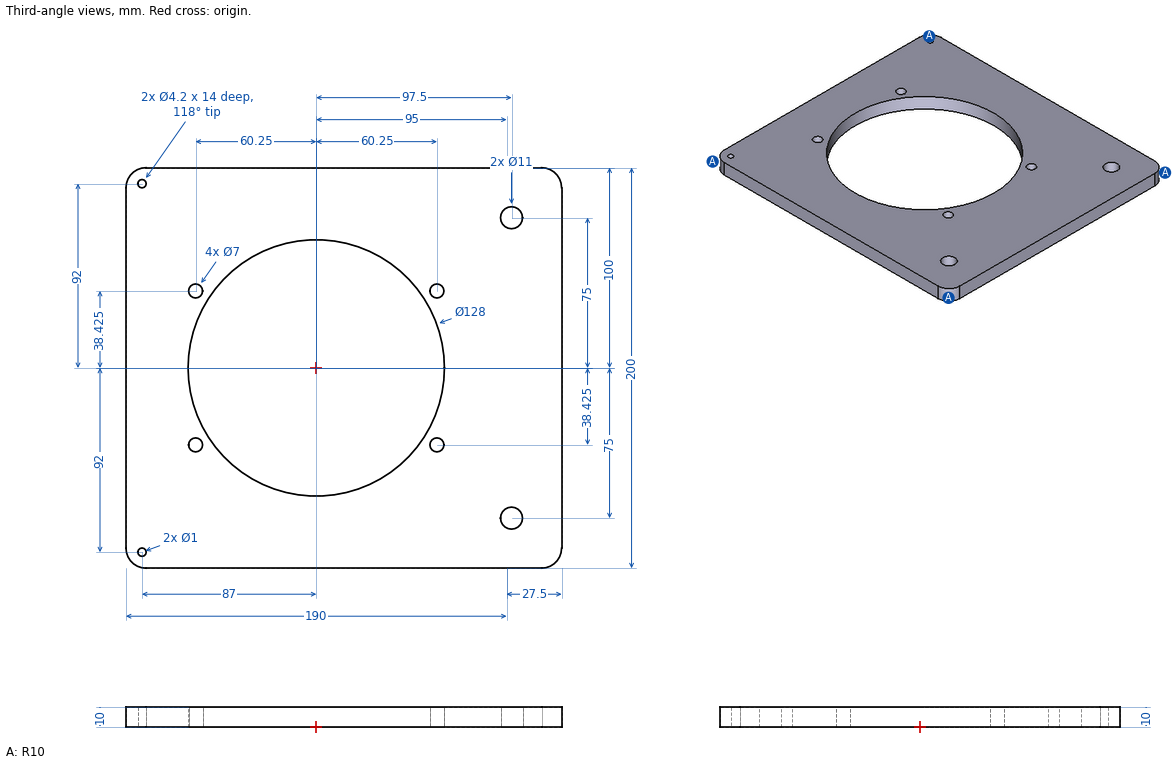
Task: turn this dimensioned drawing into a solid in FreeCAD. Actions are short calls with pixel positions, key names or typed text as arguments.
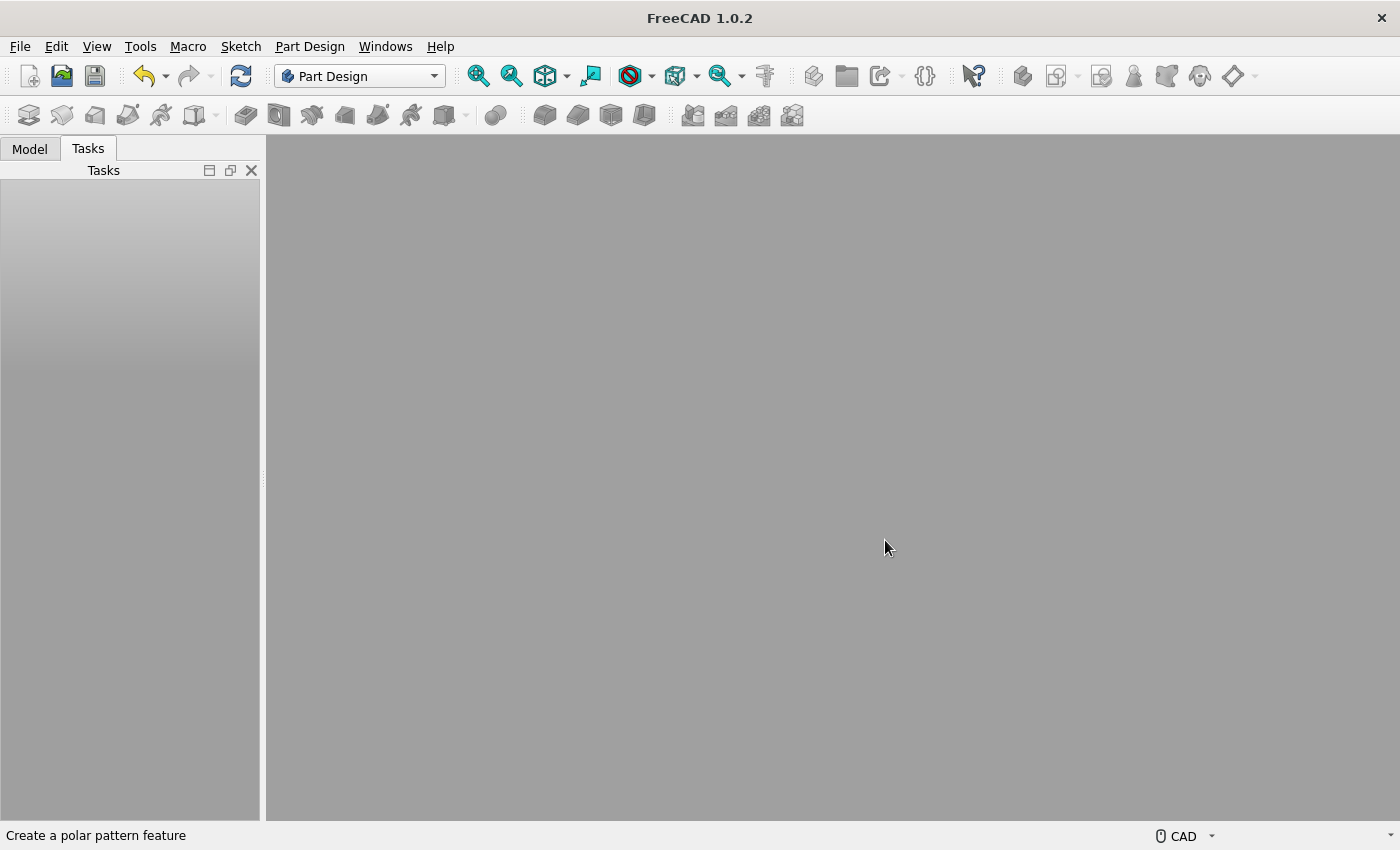
click(29, 76)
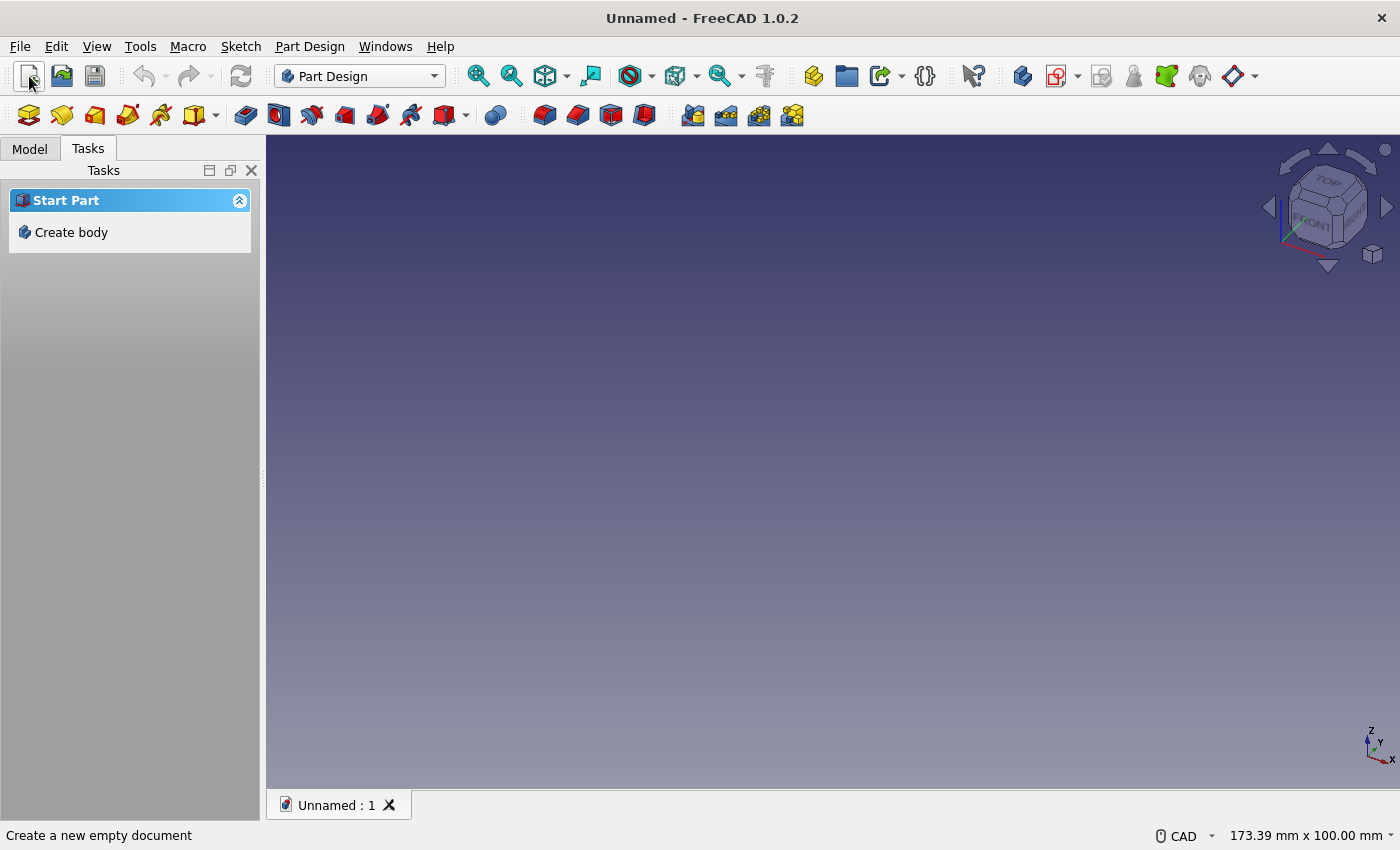
click(1056, 76)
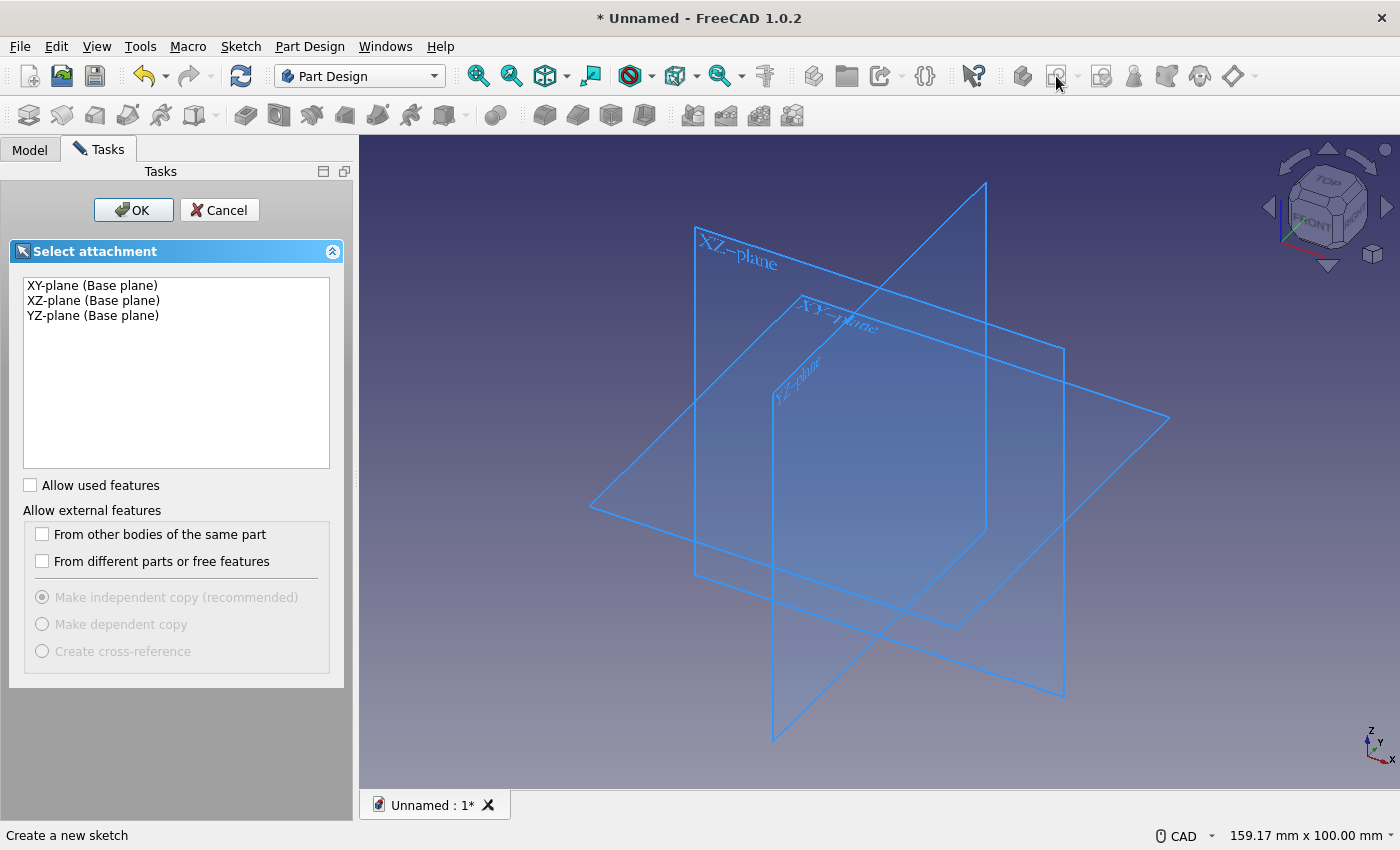
click(84, 286)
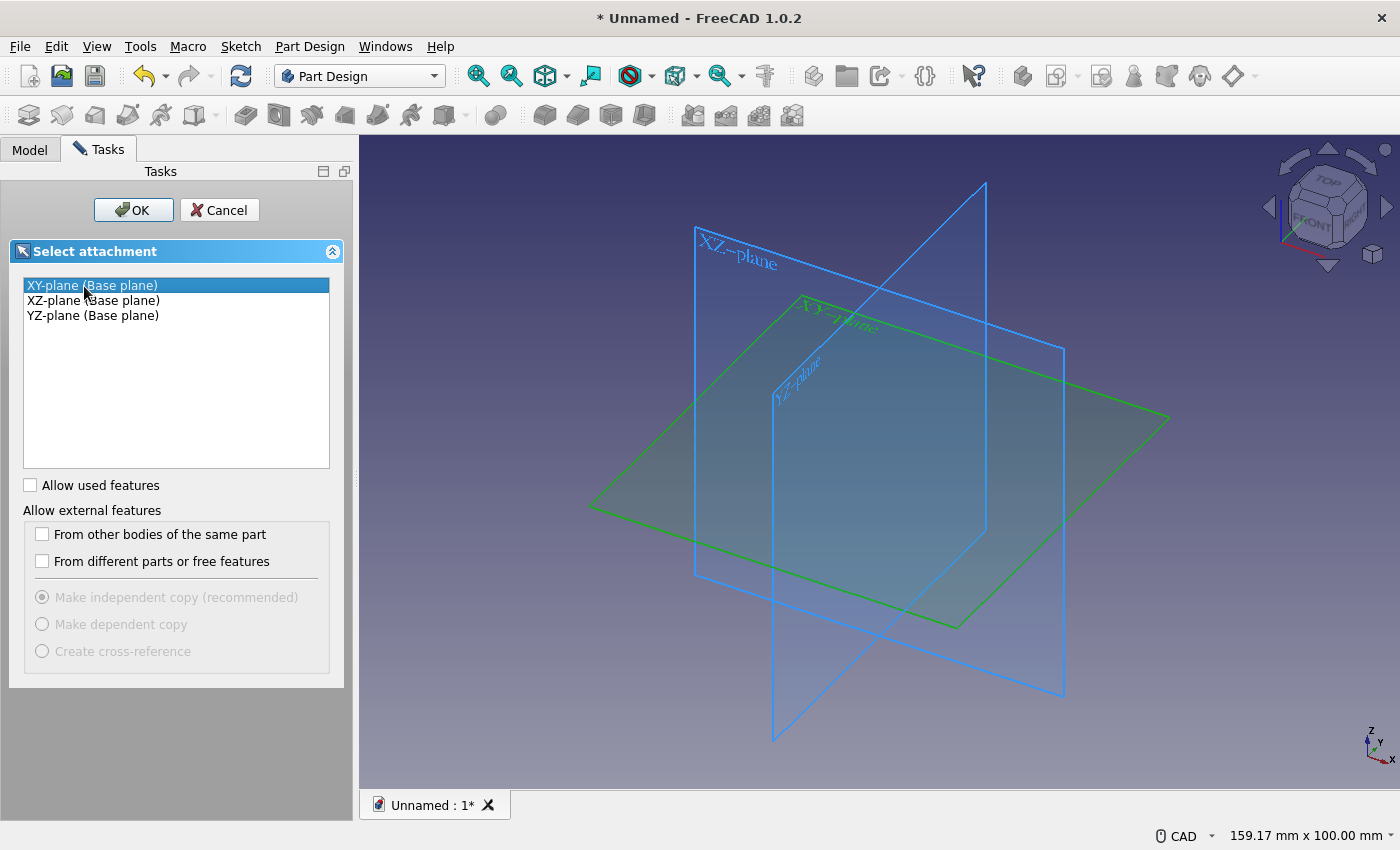
click(134, 210)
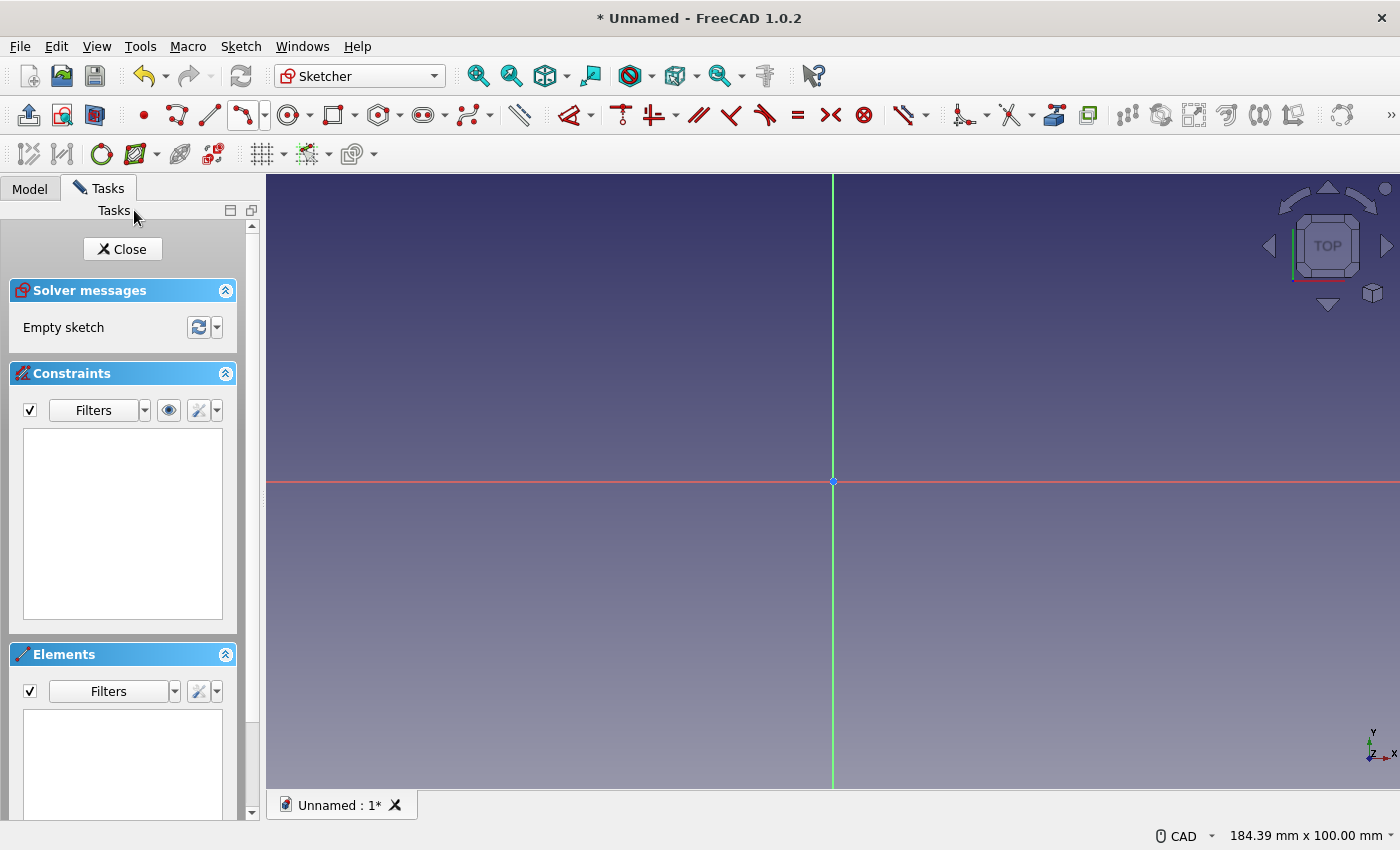
scroll(735, 482, down, 6)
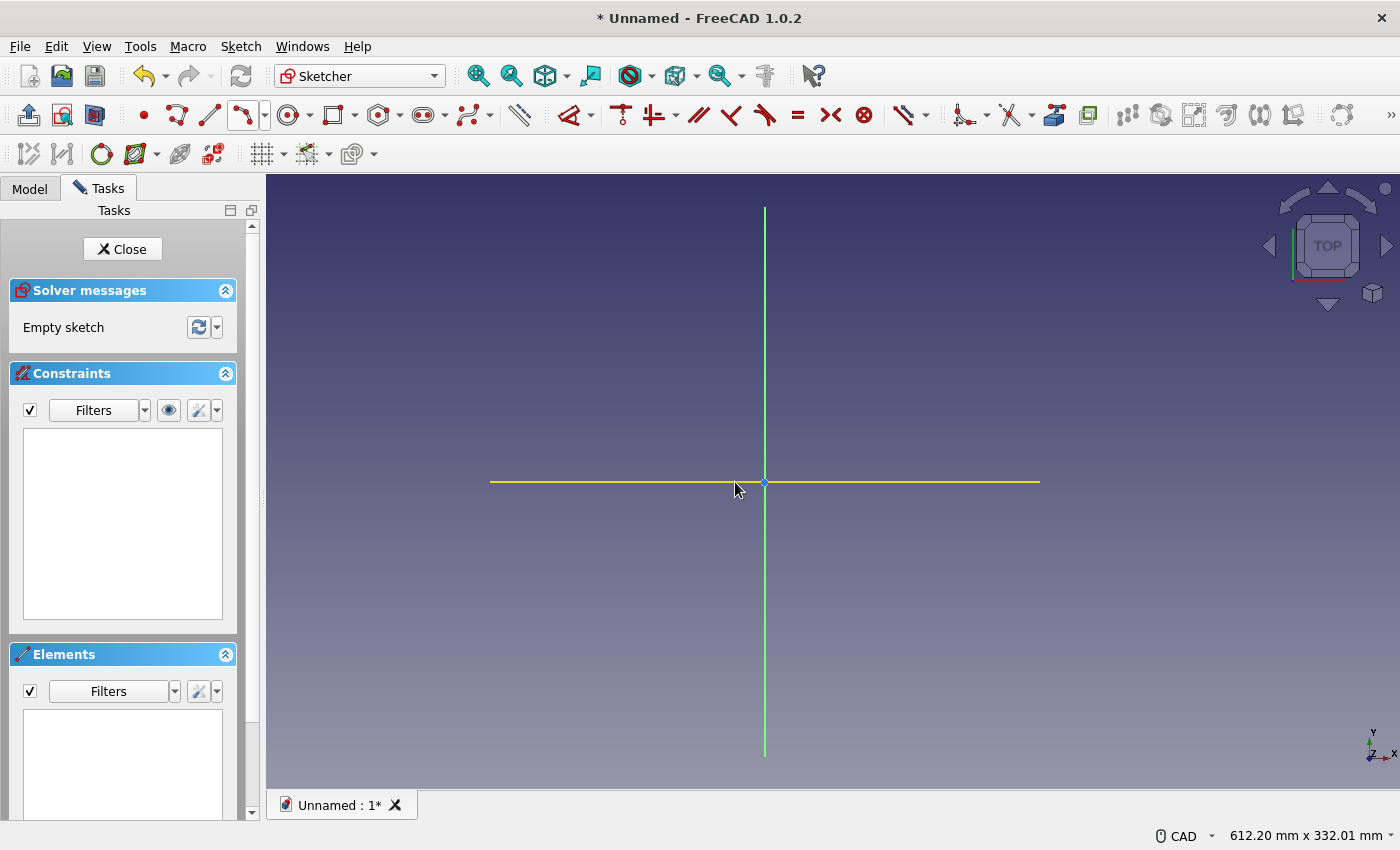
key(g)
key(v)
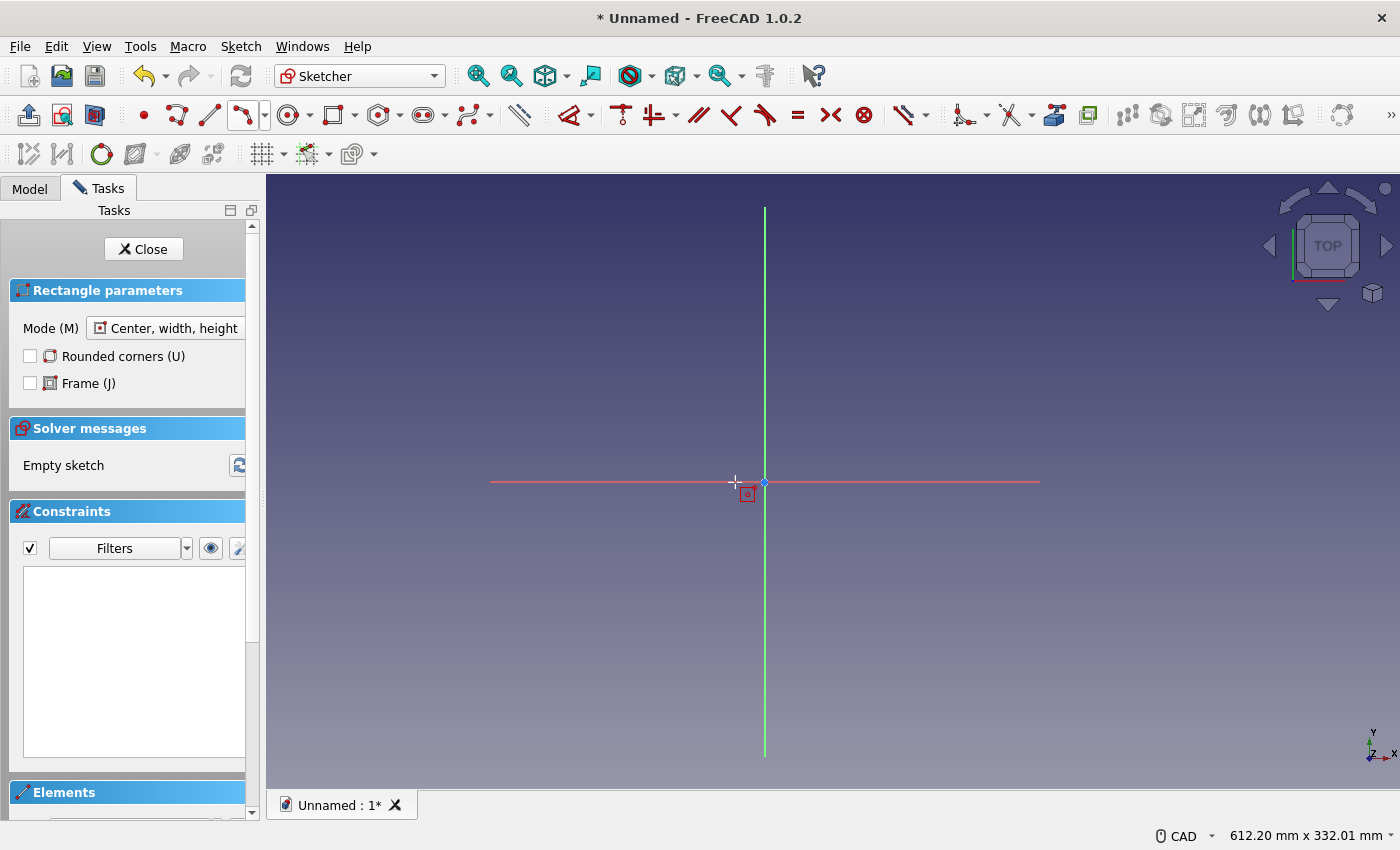
click(765, 482)
move(941, 297)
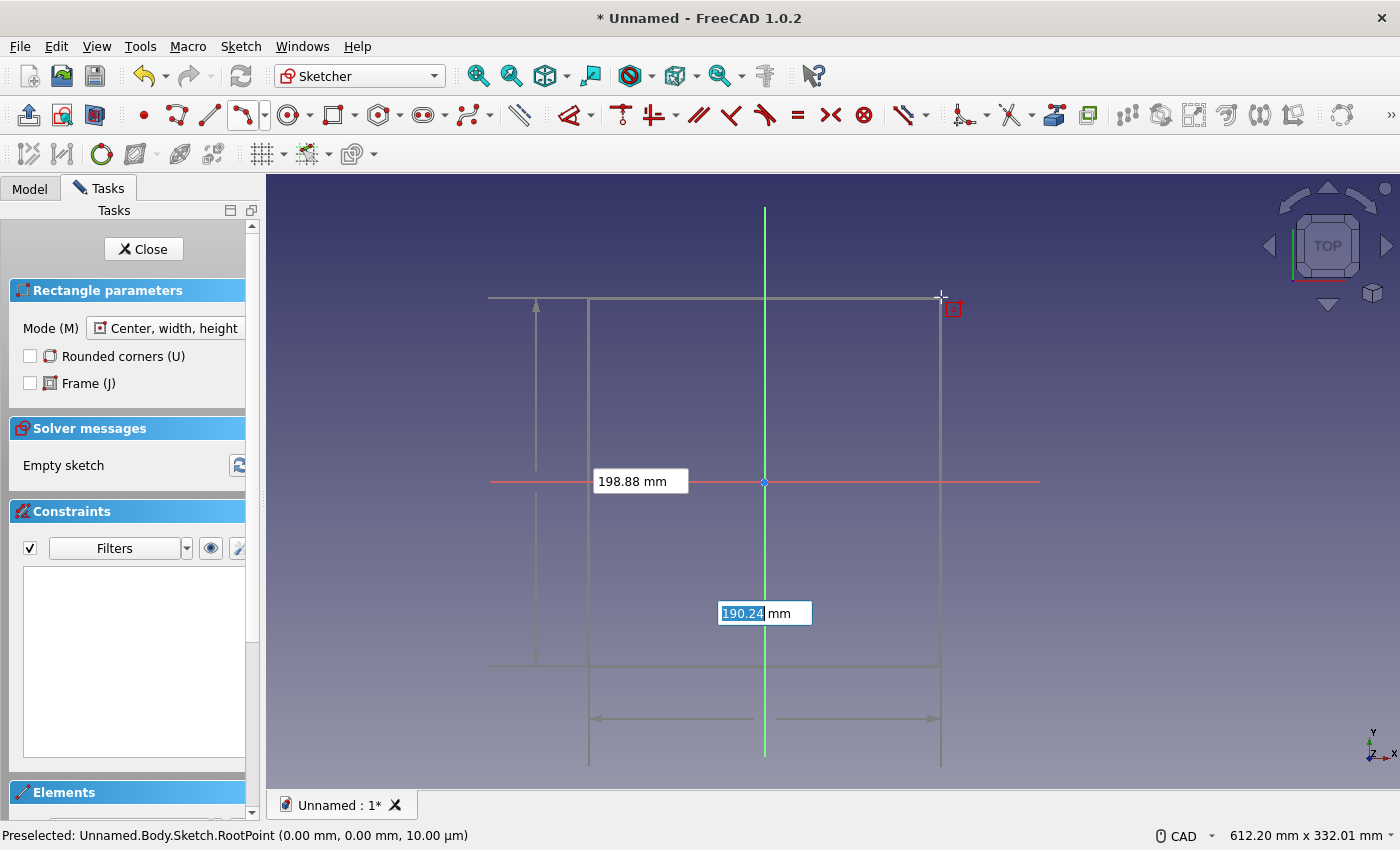
text(190)
key(Tab)
text(200)
key(Return)
key(Escape)